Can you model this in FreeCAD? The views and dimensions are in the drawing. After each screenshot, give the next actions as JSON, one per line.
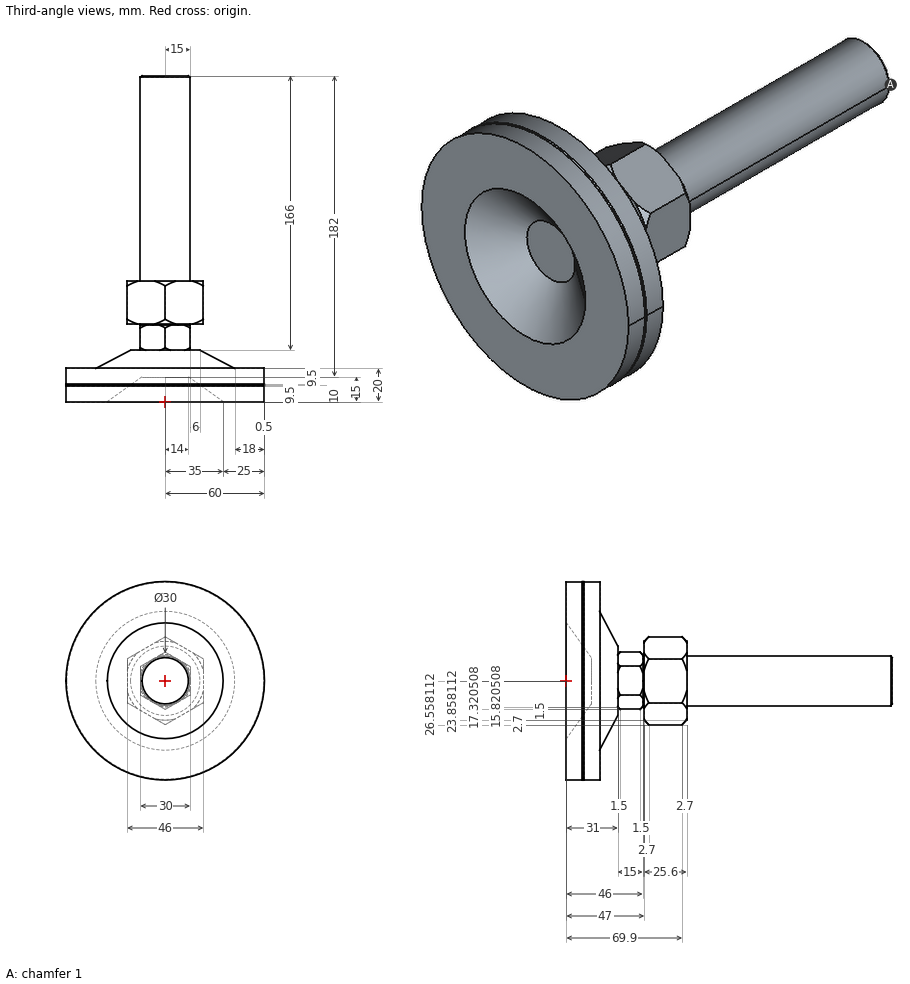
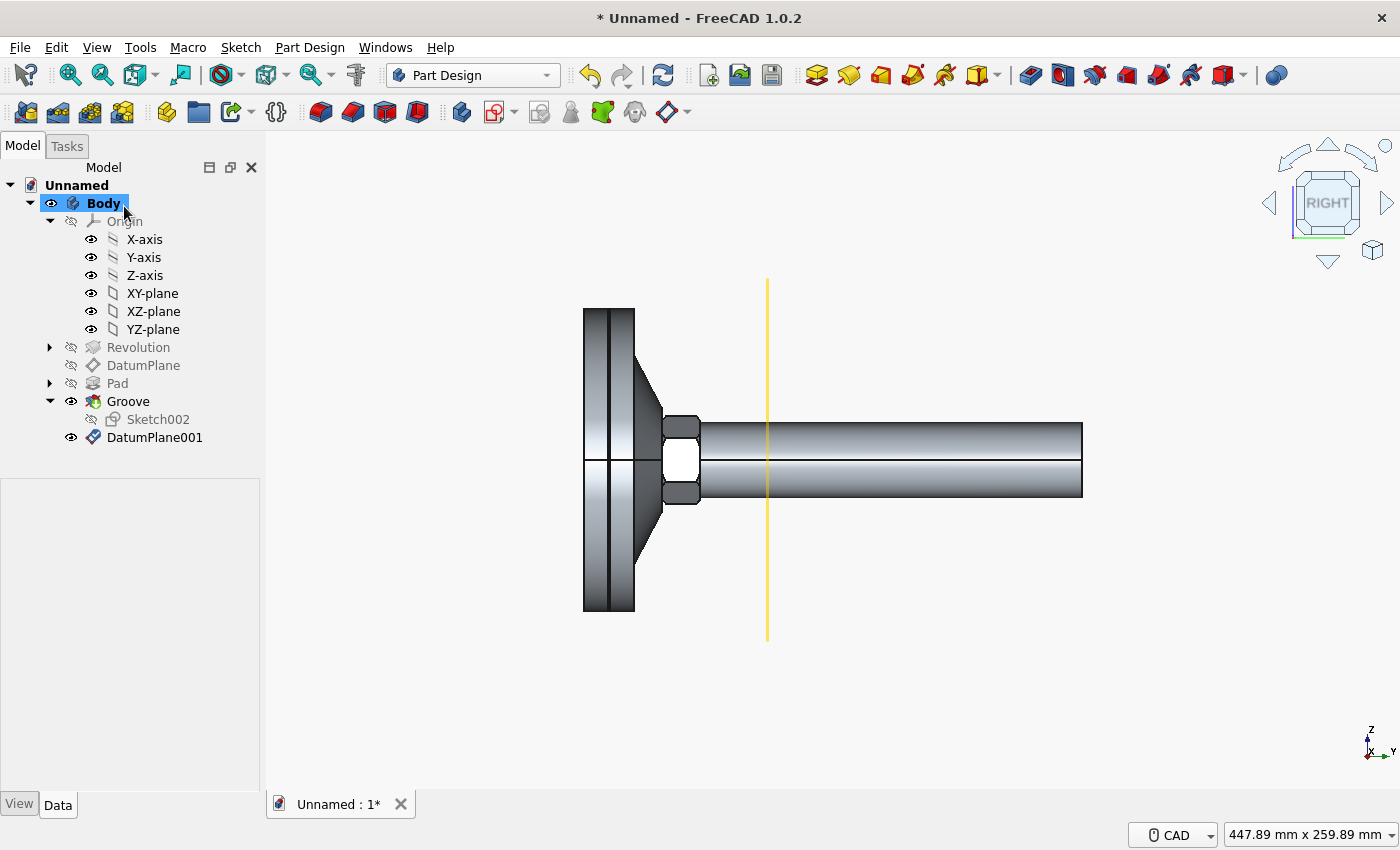
{"action": "left_click", "coordinate": [116, 437]}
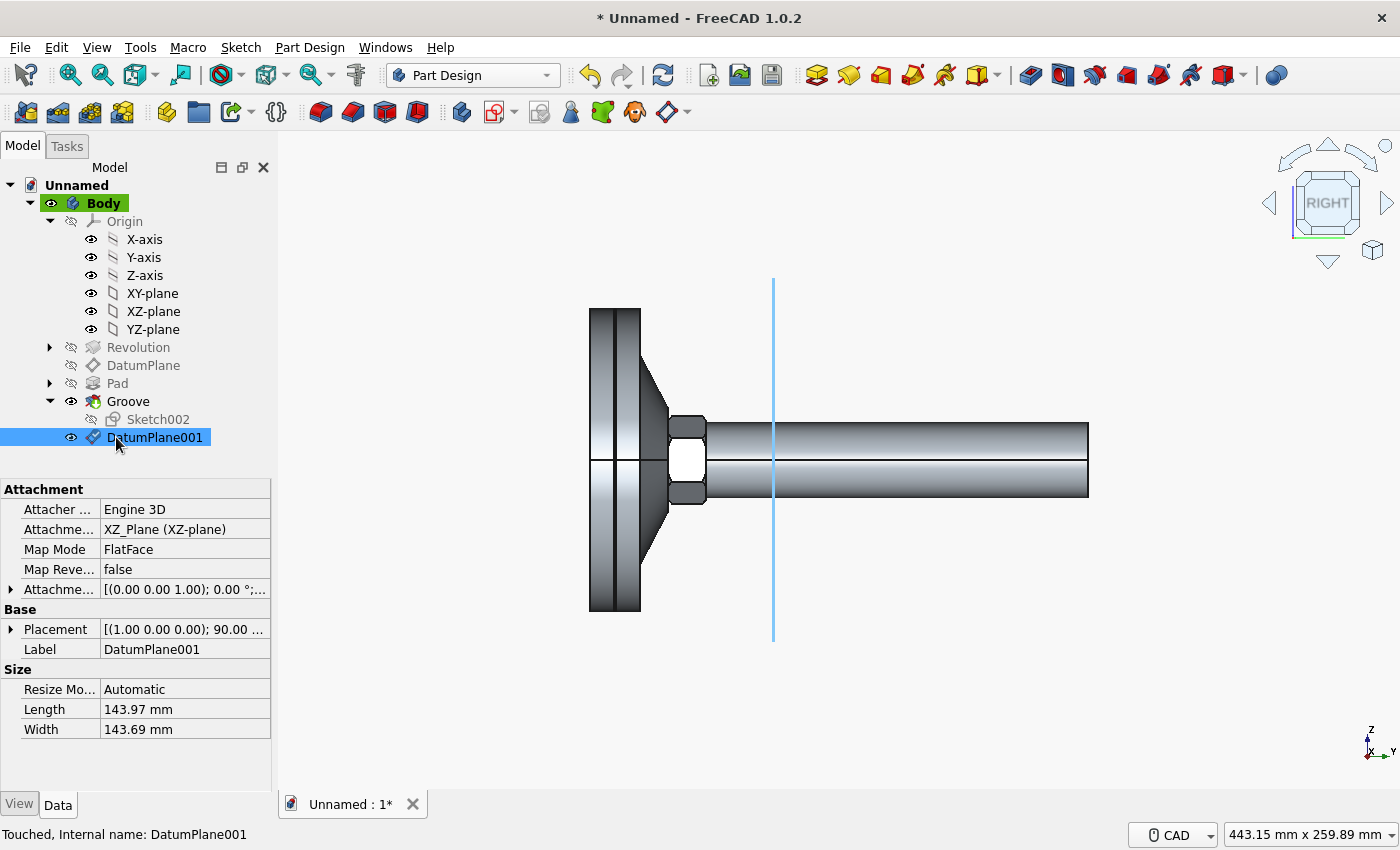
{"action": "left_click", "coordinate": [494, 112]}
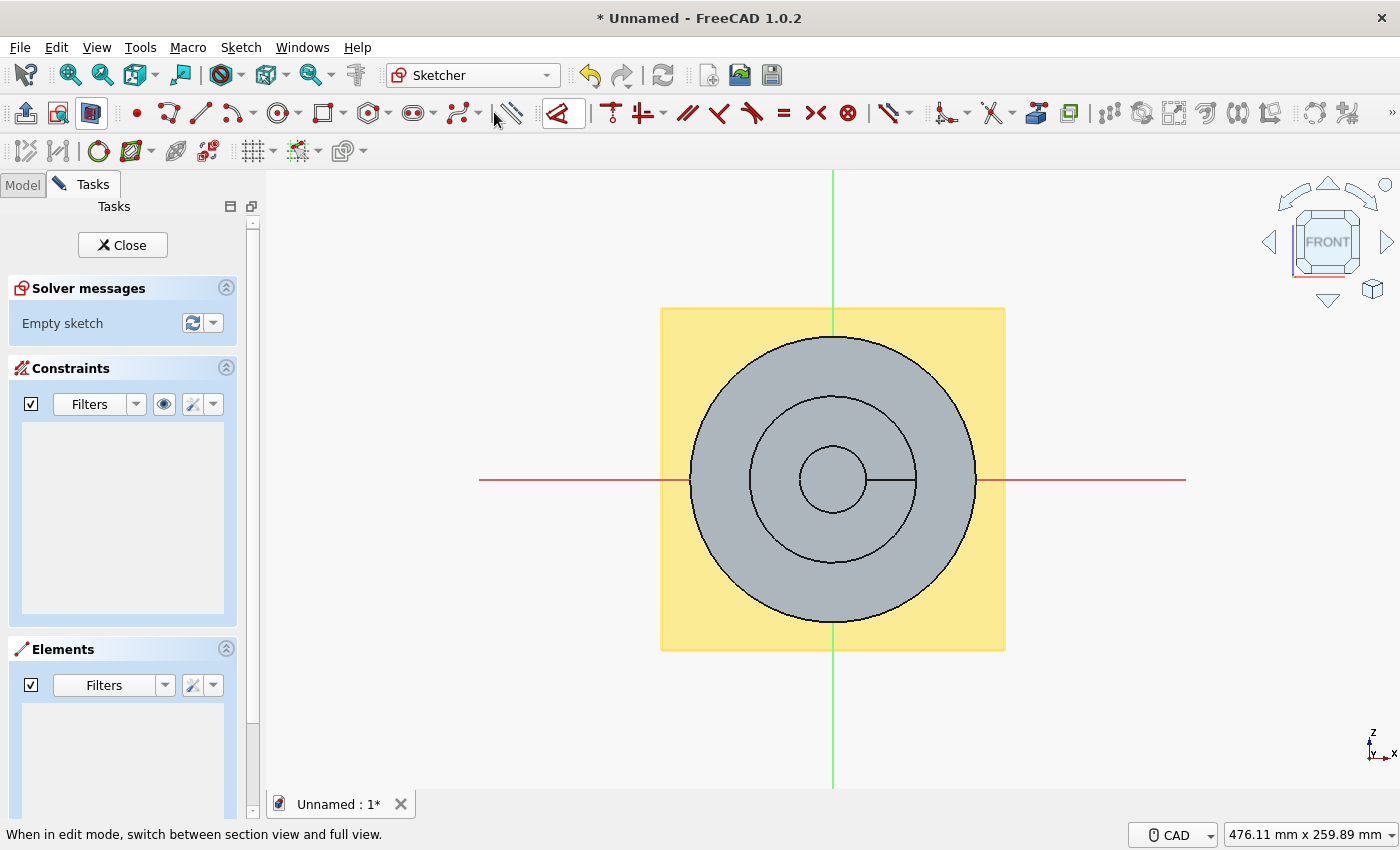
{"action": "key", "text": "q s"}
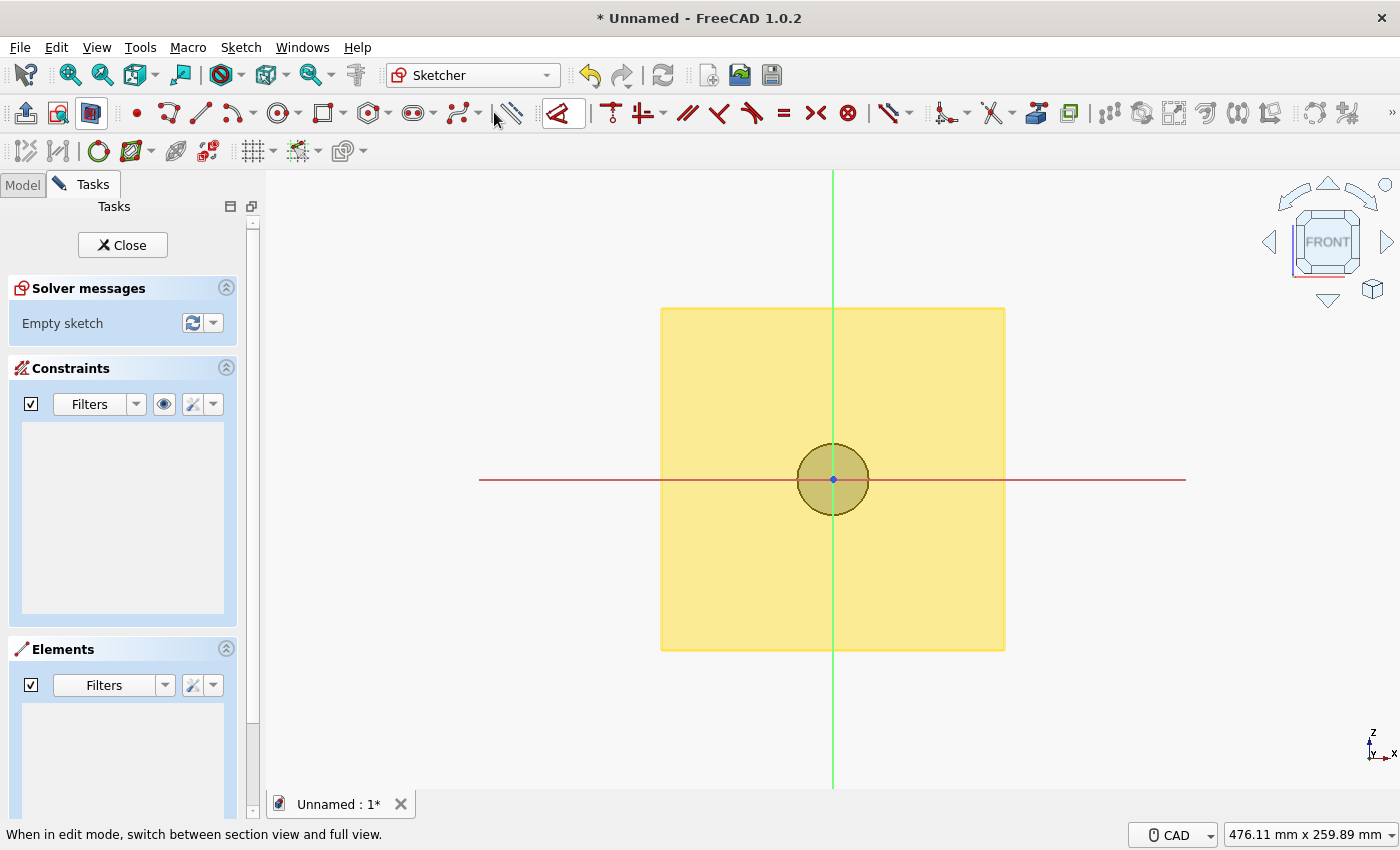
{"action": "scroll", "coordinate": [863, 480], "scroll_direction": "up", "scroll_amount": 6}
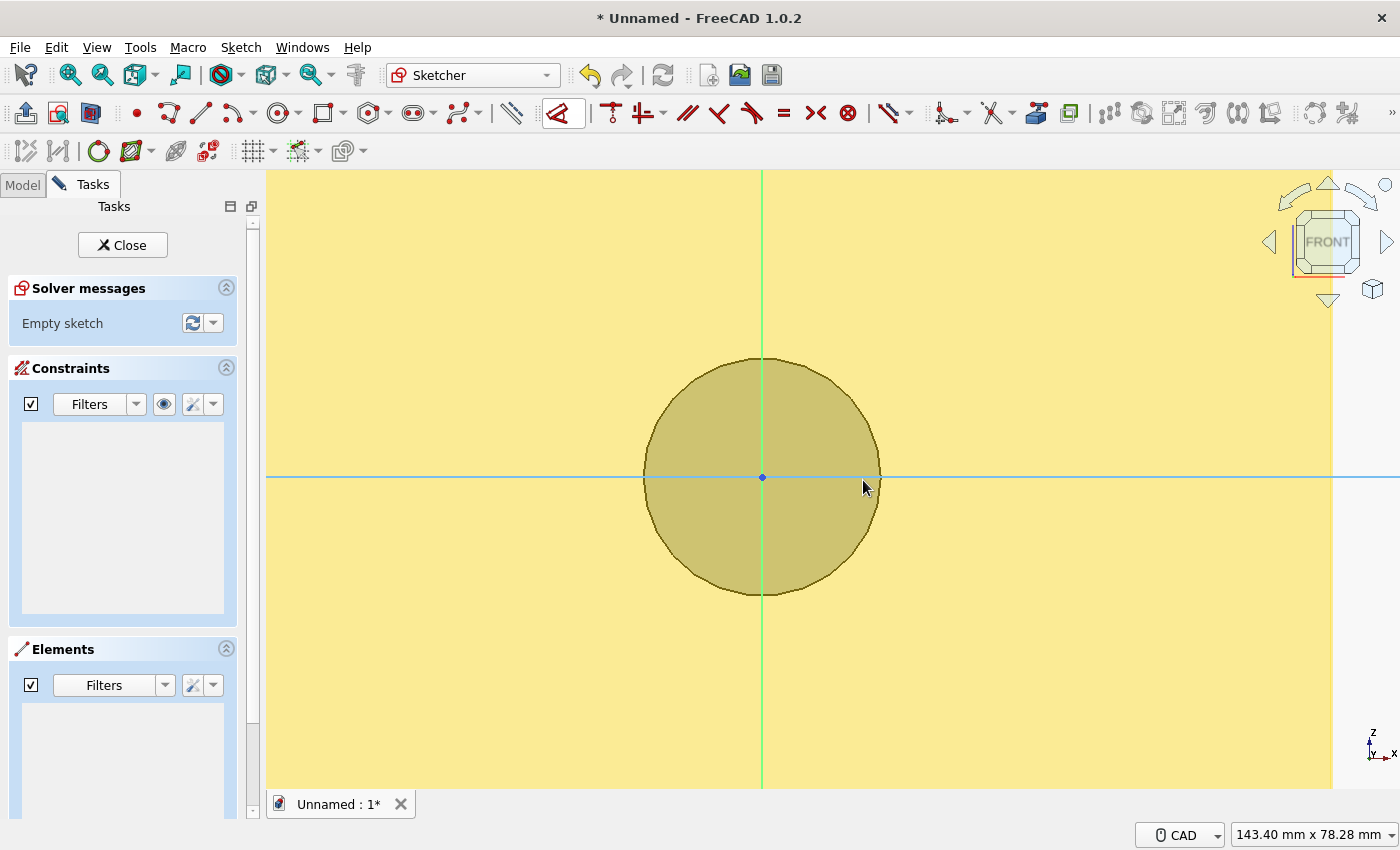
{"action": "key", "text": "g p 6"}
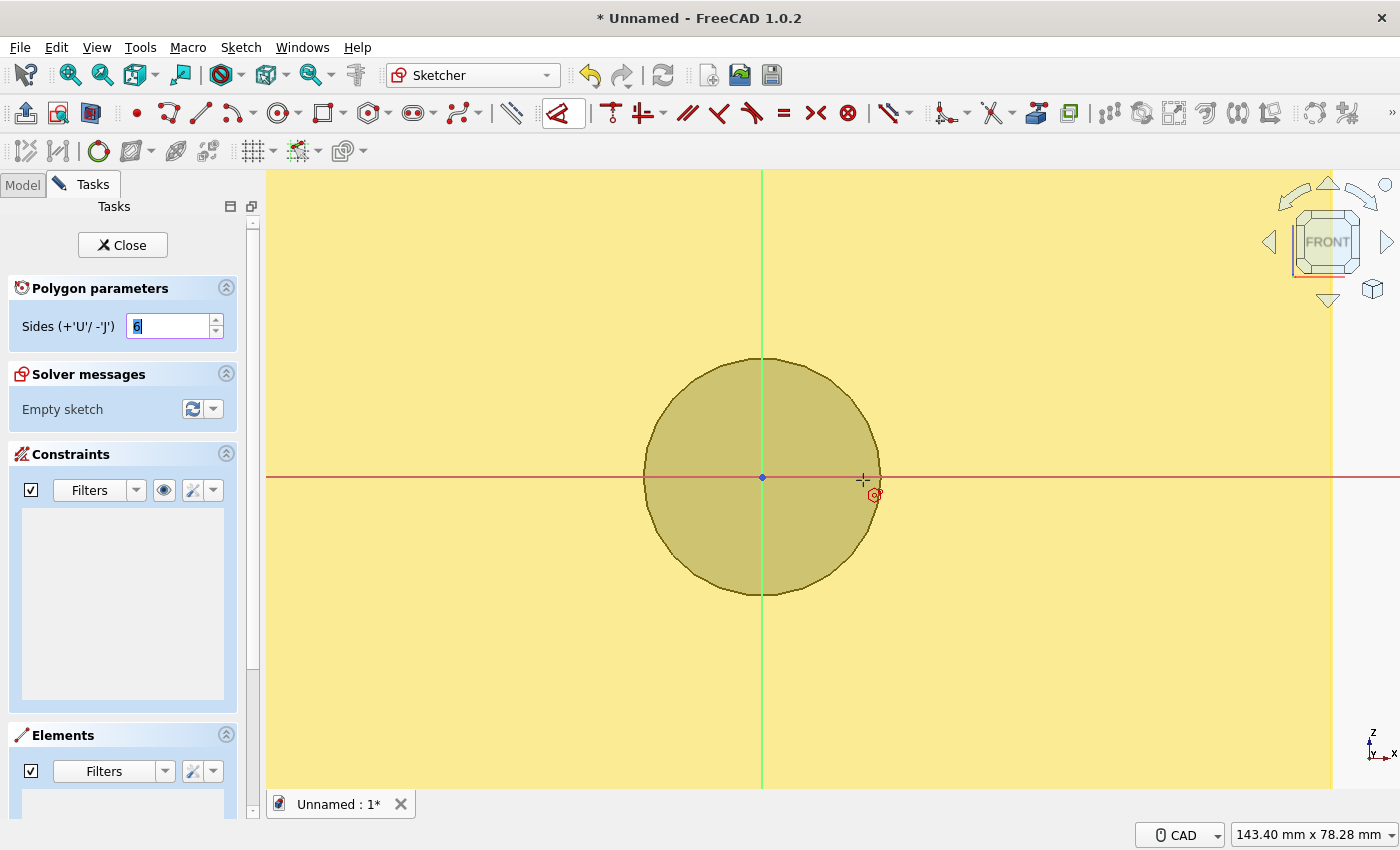
{"action": "left_click", "coordinate": [762, 477]}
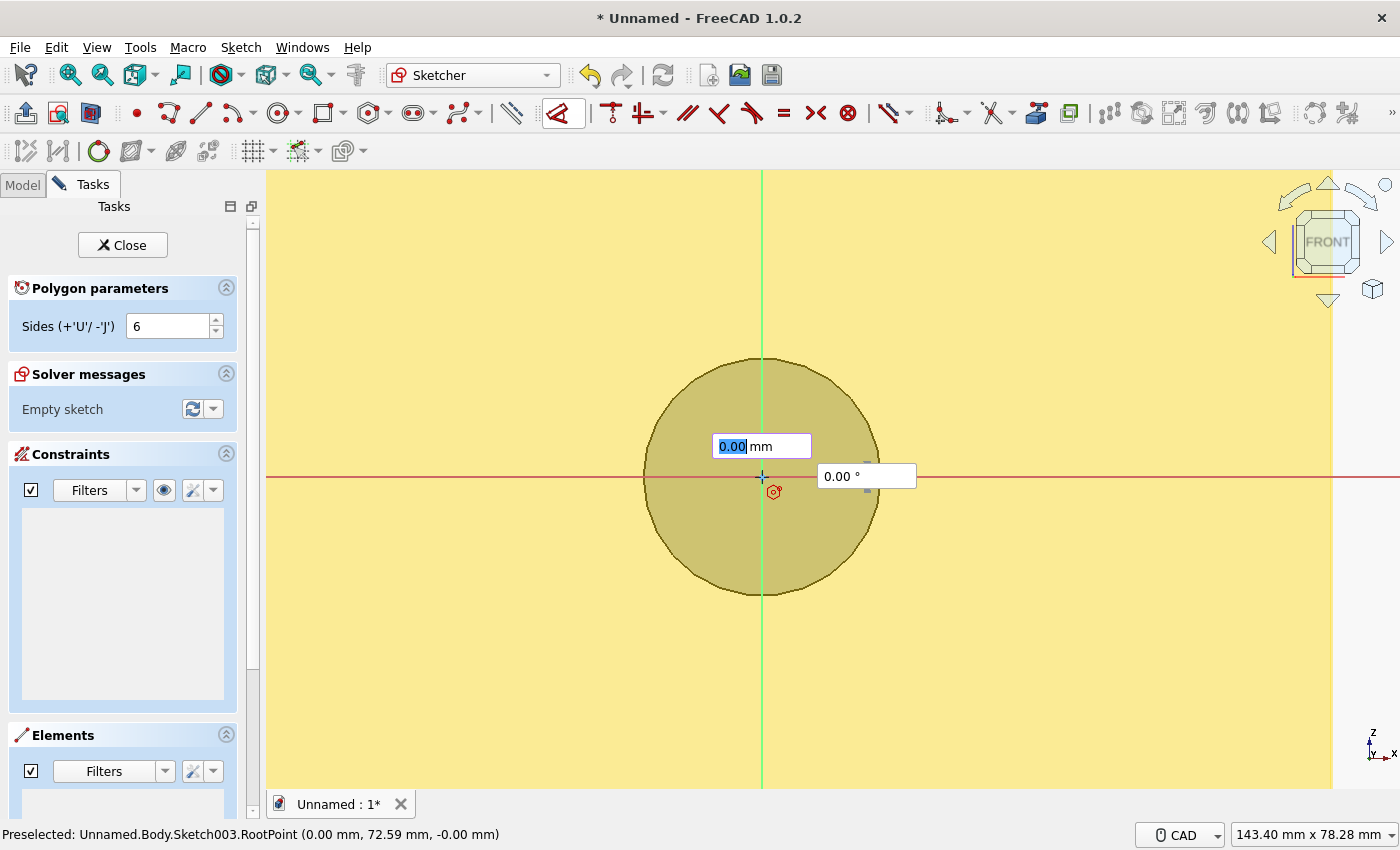
{"action": "left_click", "coordinate": [762, 267]}
{"action": "right_click", "coordinate": [762, 267]}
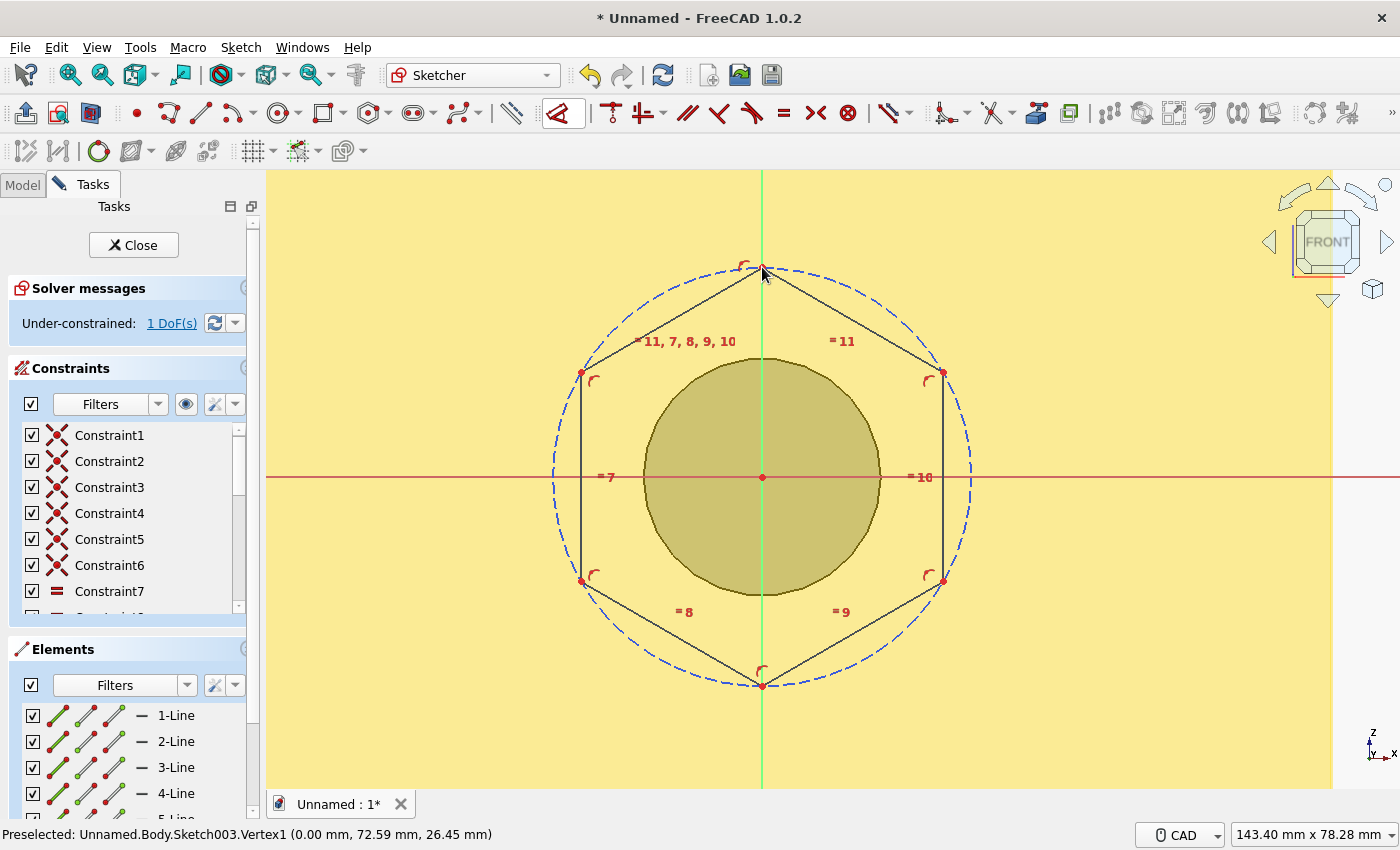
{"action": "key", "text": "g c"}